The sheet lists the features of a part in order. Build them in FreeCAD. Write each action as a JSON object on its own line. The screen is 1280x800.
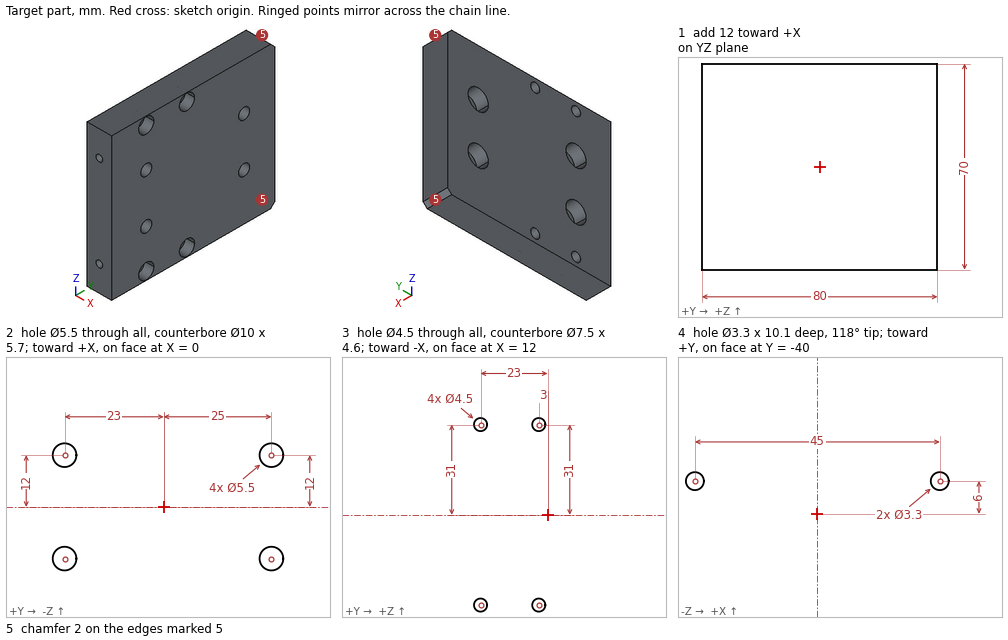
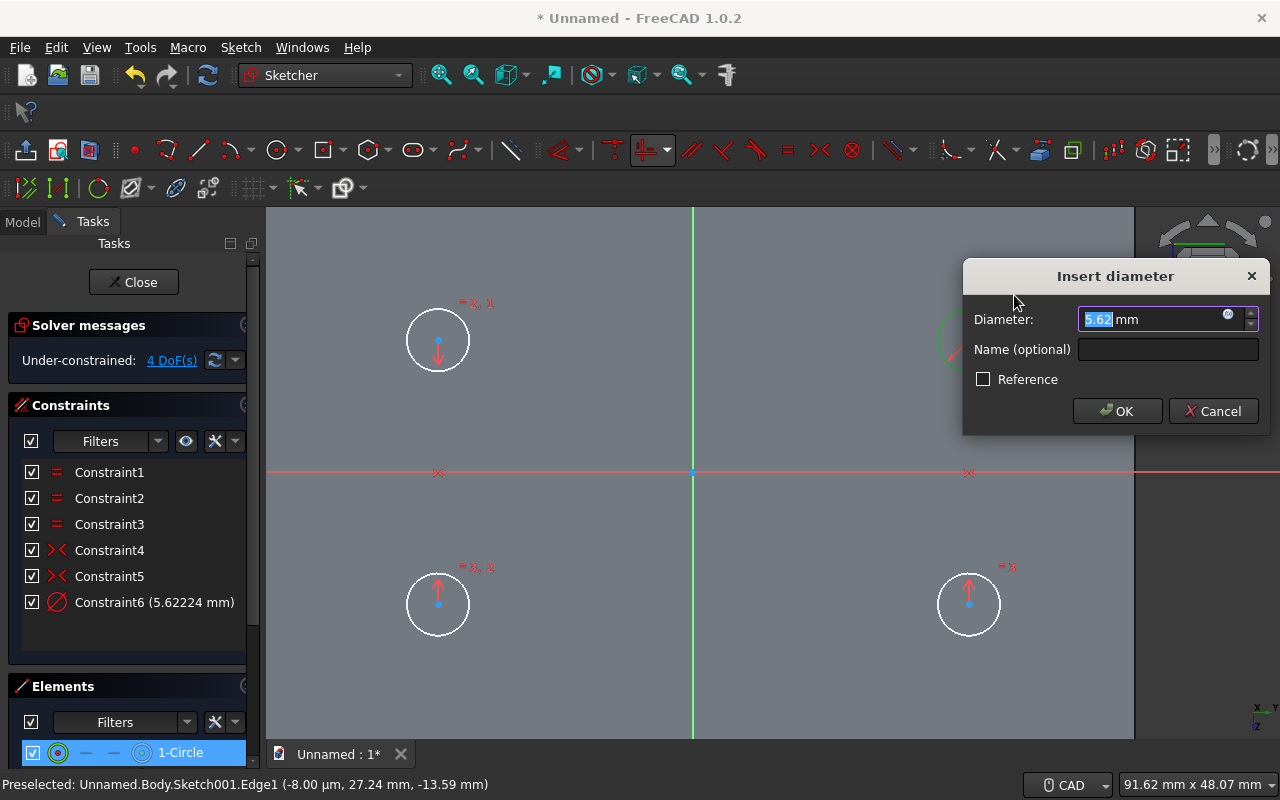
{"action": "type", "text": "5.5"}
{"action": "key", "text": "Return"}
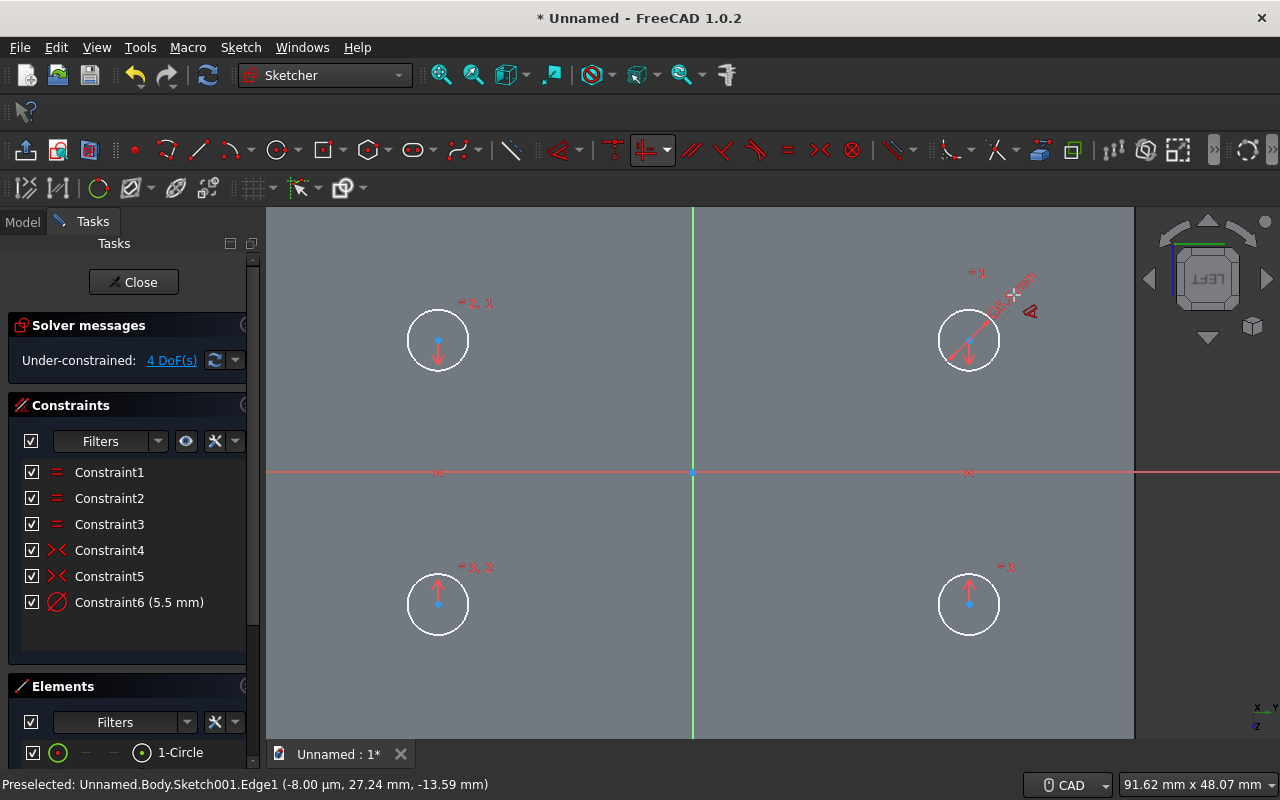
{"action": "left_click", "coordinate": [969, 340]}
{"action": "left_click", "coordinate": [831, 306]}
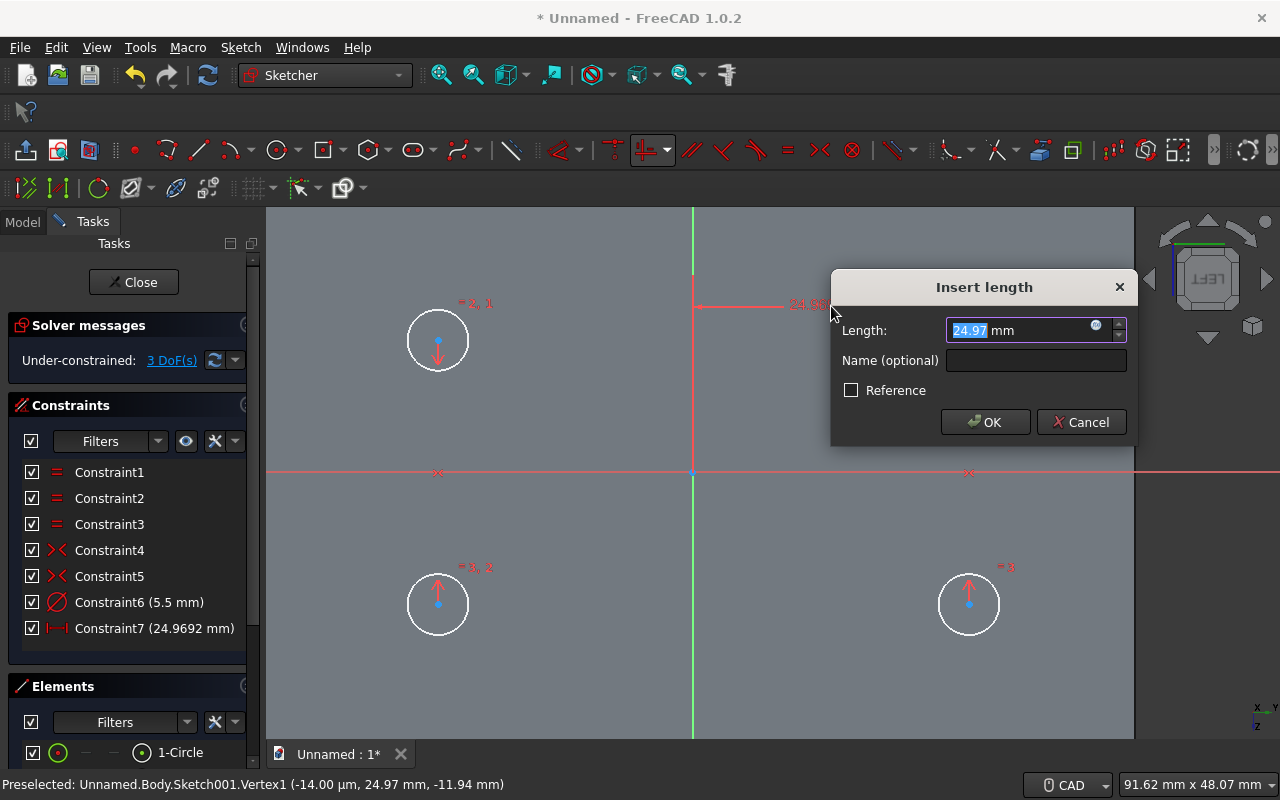
{"action": "type", "text": "25"}
{"action": "key", "text": "Return"}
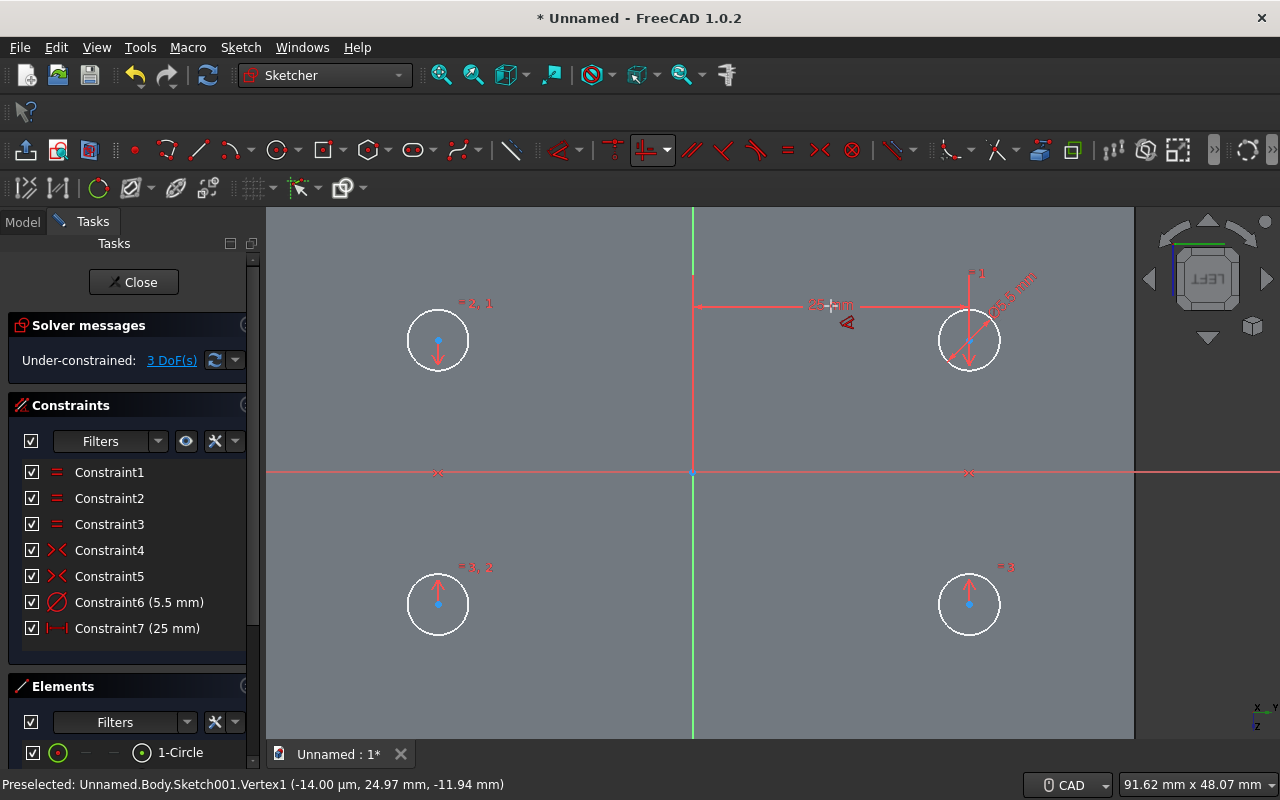
{"action": "left_click", "coordinate": [969, 340]}
{"action": "left_click", "coordinate": [1003, 406]}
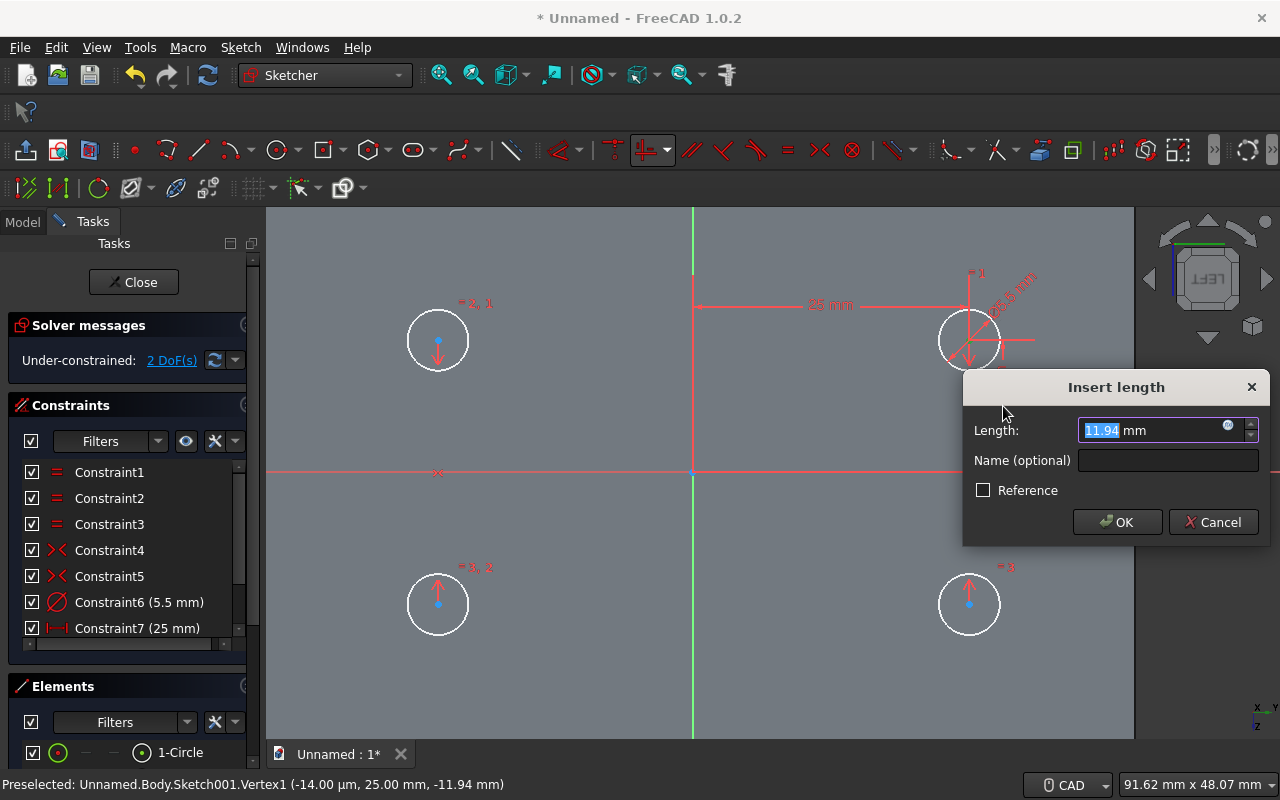
{"action": "type", "text": "12"}
{"action": "key", "text": "Return"}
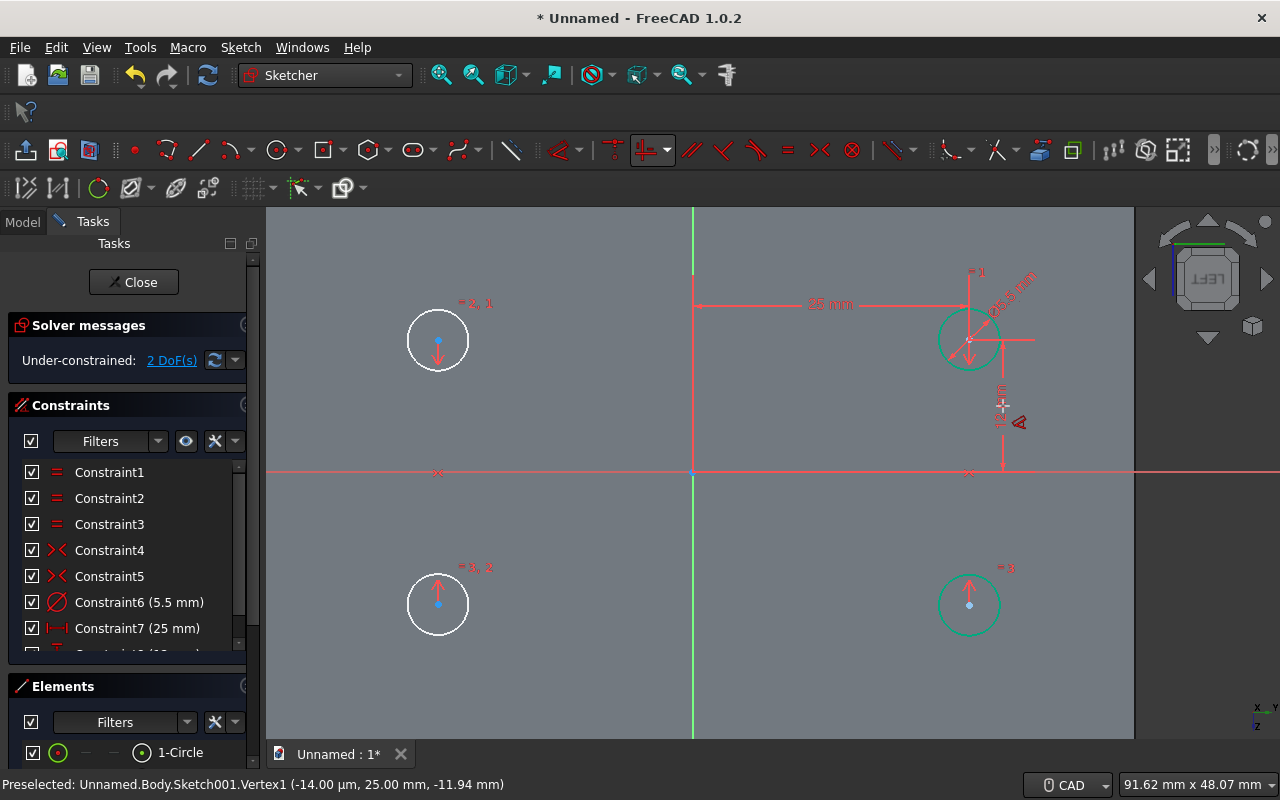
{"action": "left_click", "coordinate": [438, 340]}
{"action": "left_click", "coordinate": [565, 306]}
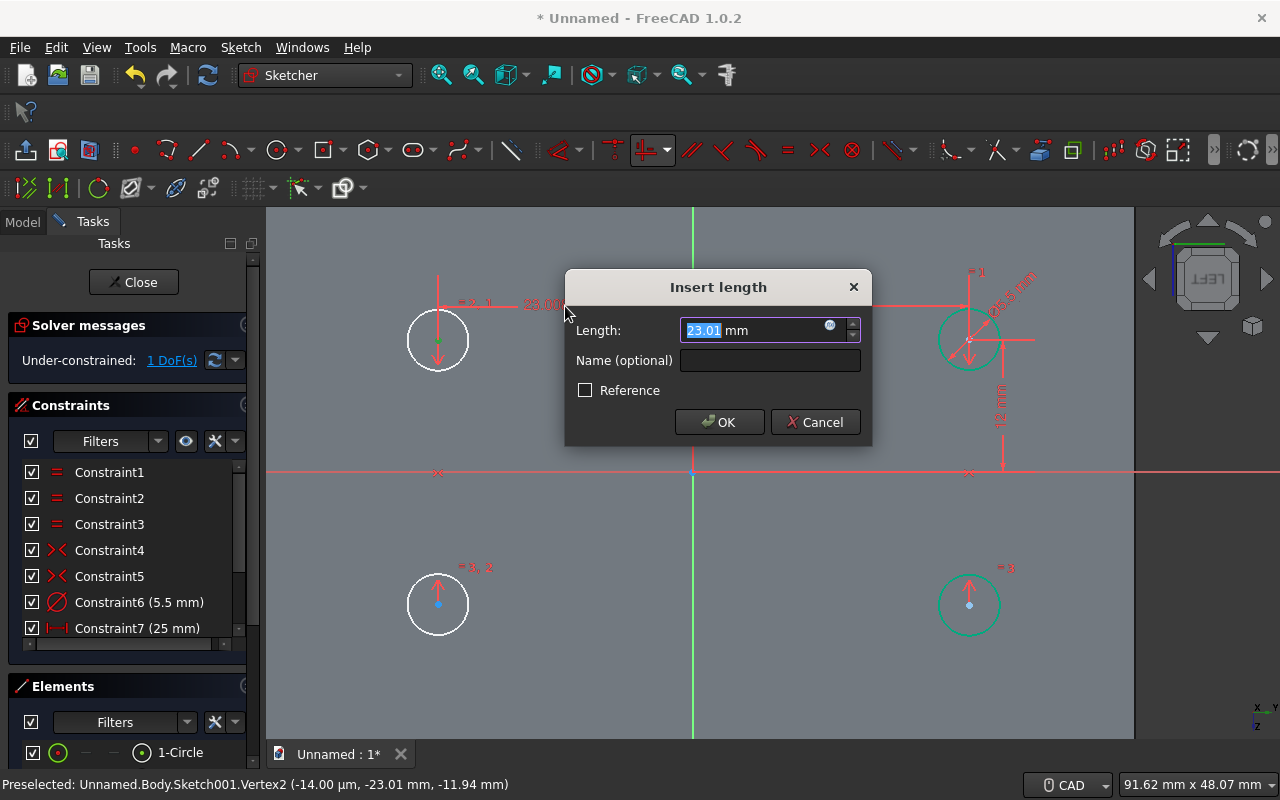
{"action": "type", "text": "23"}
{"action": "key", "text": "Return"}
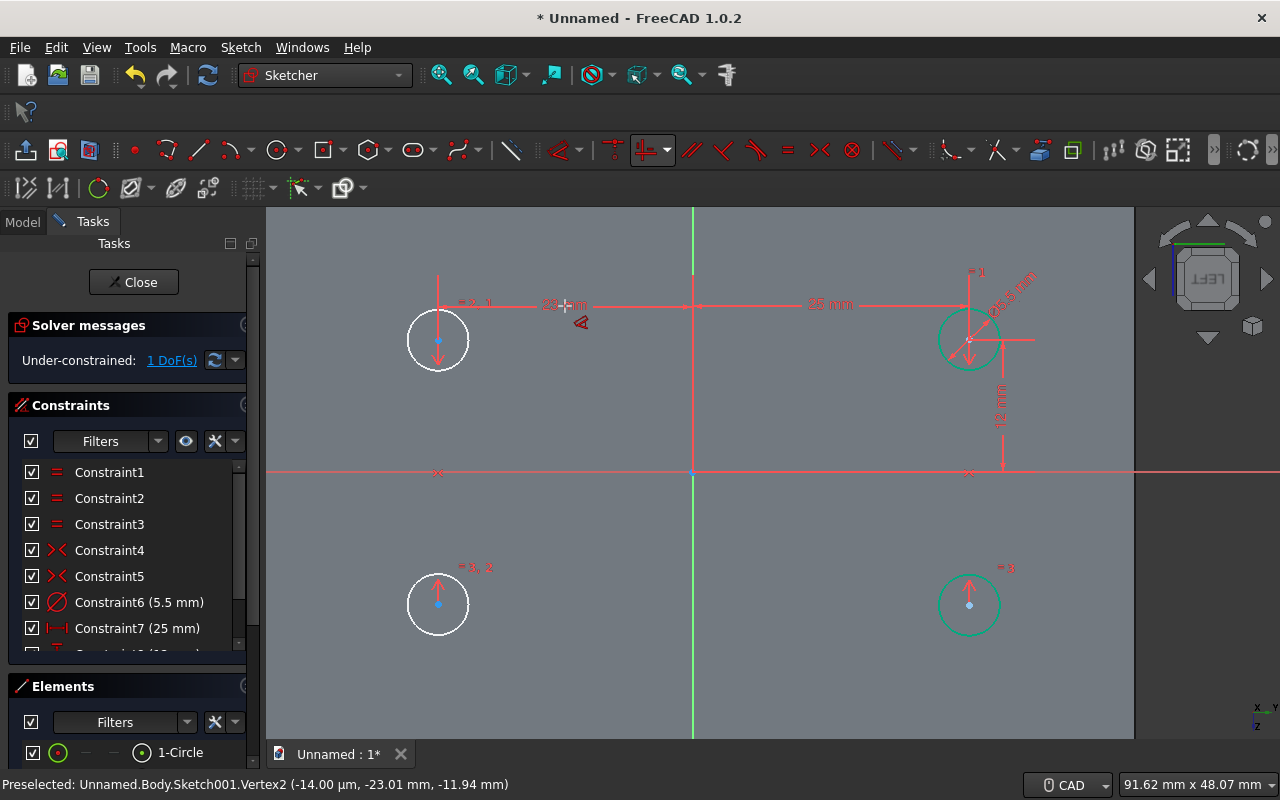
{"action": "left_click", "coordinate": [438, 340]}
{"action": "left_click", "coordinate": [404, 406]}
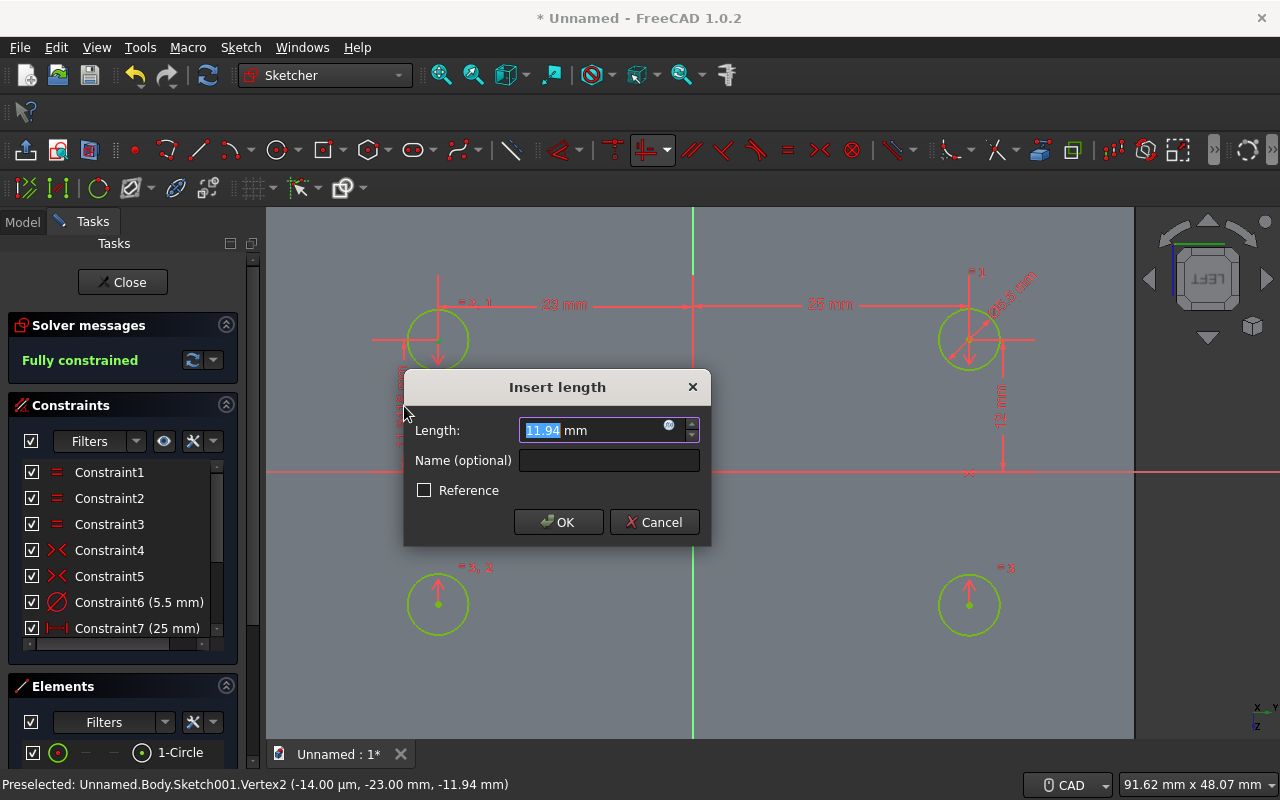
{"action": "type", "text": "12"}
{"action": "key", "text": "Return"}
{"action": "key", "text": "Escape"}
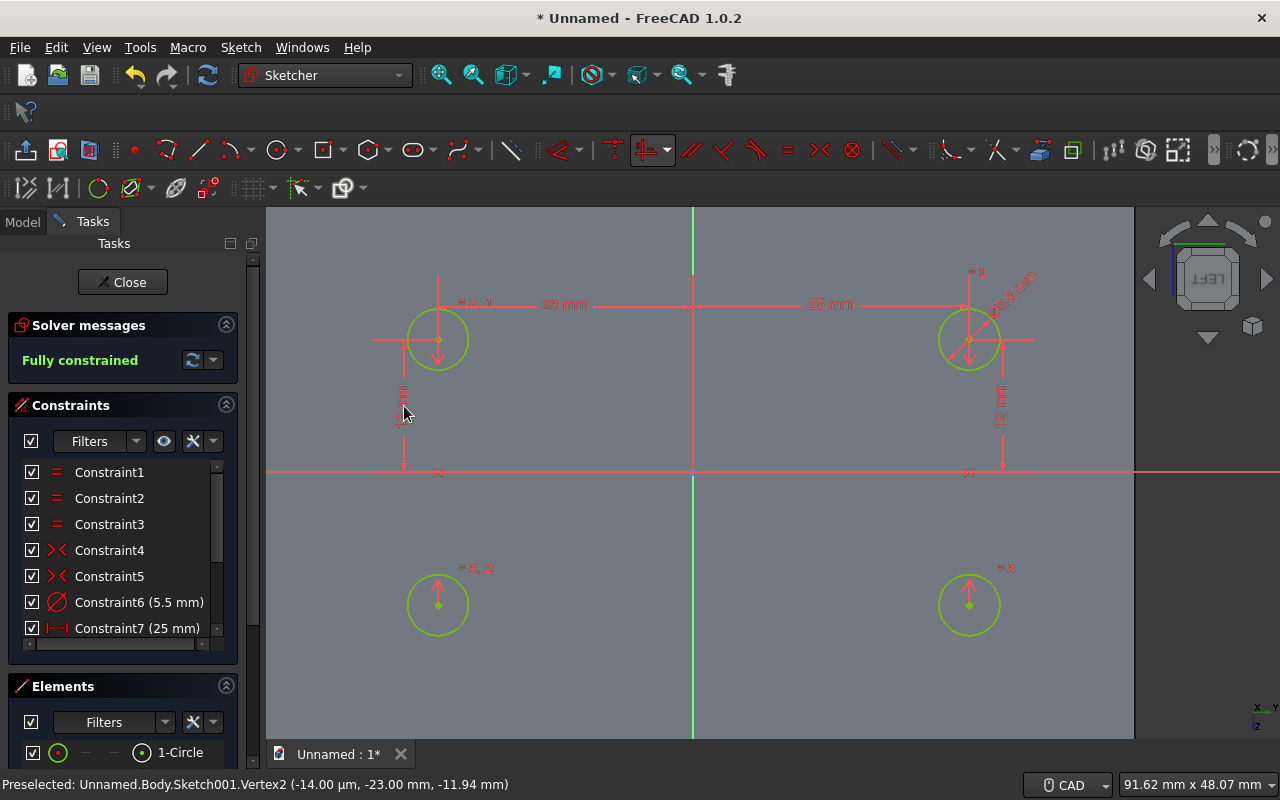
{"action": "left_click", "coordinate": [123, 282]}